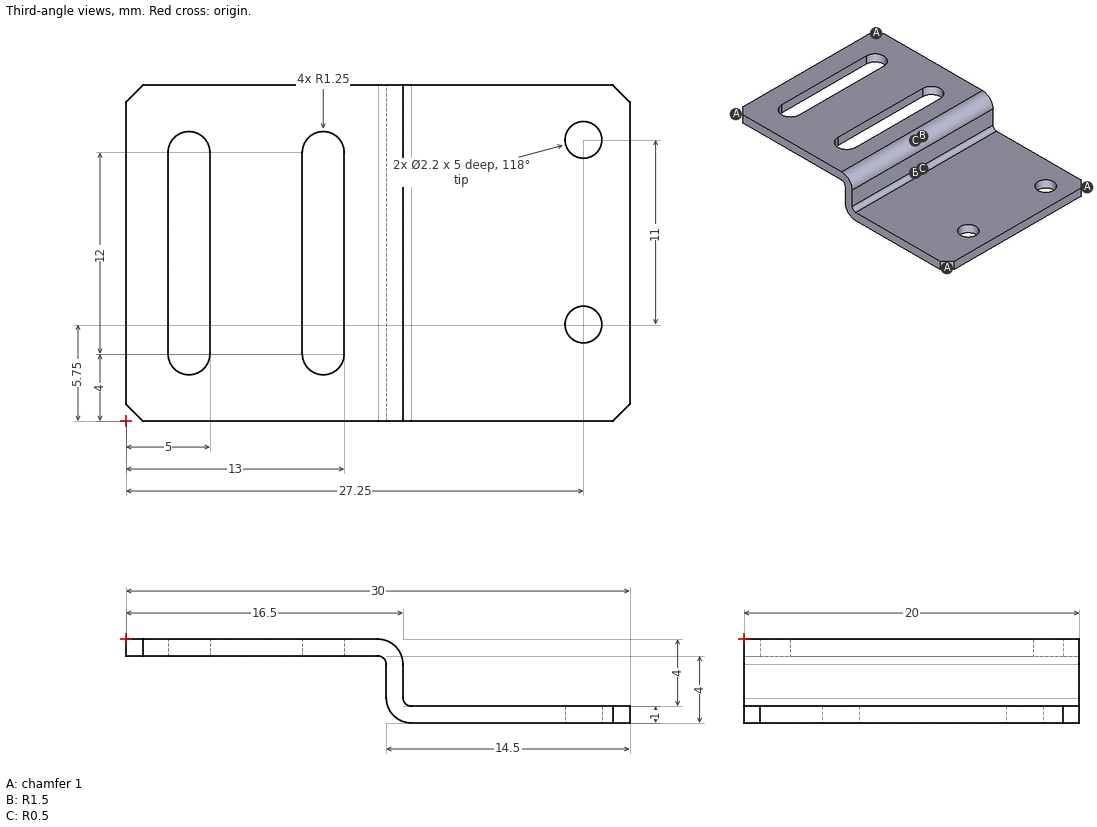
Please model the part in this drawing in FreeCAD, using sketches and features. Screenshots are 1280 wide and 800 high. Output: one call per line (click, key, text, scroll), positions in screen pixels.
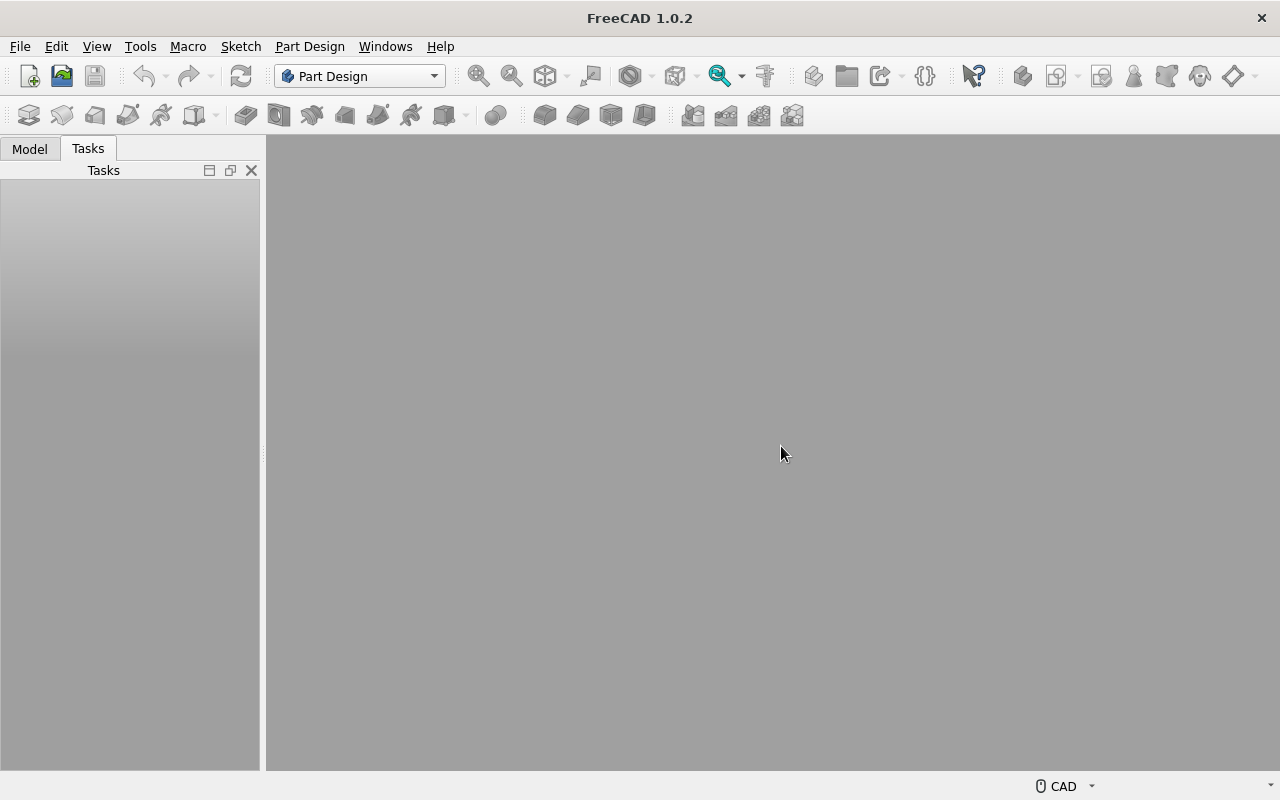
click(29, 76)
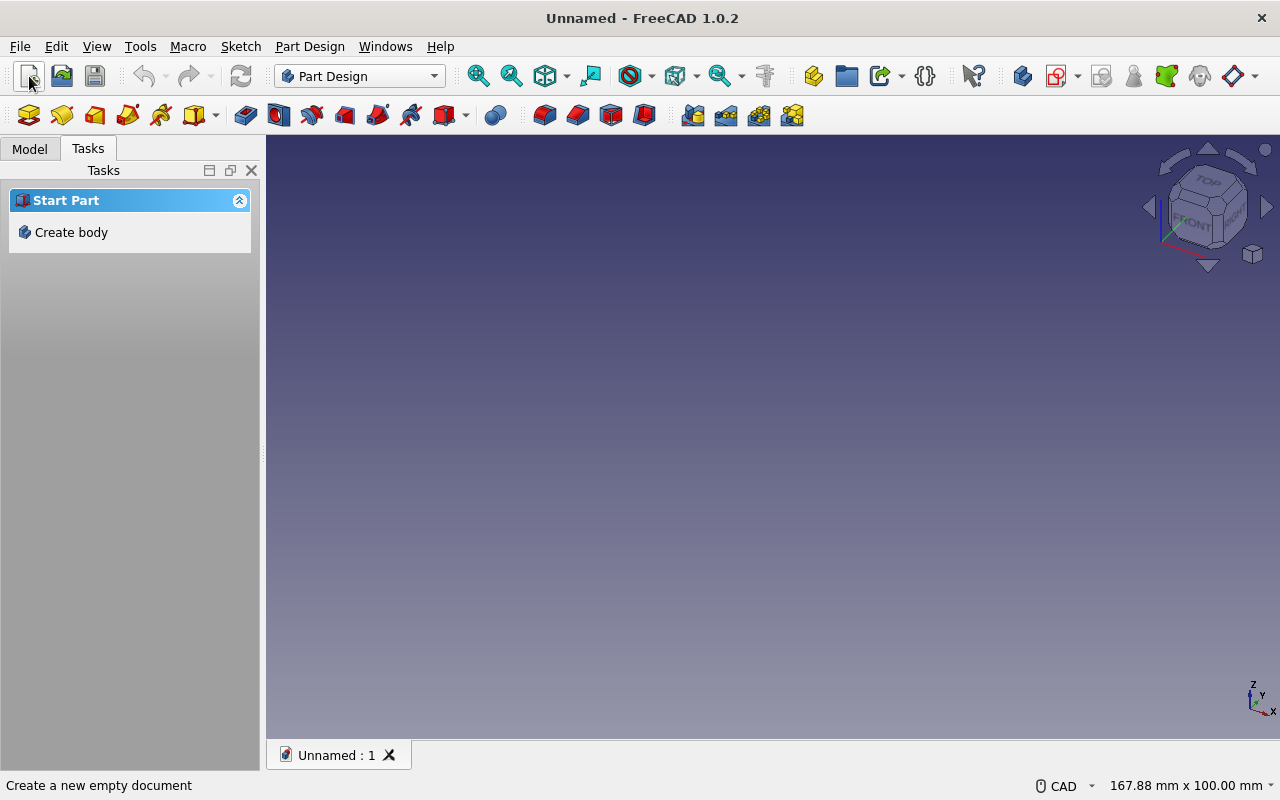
click(1056, 76)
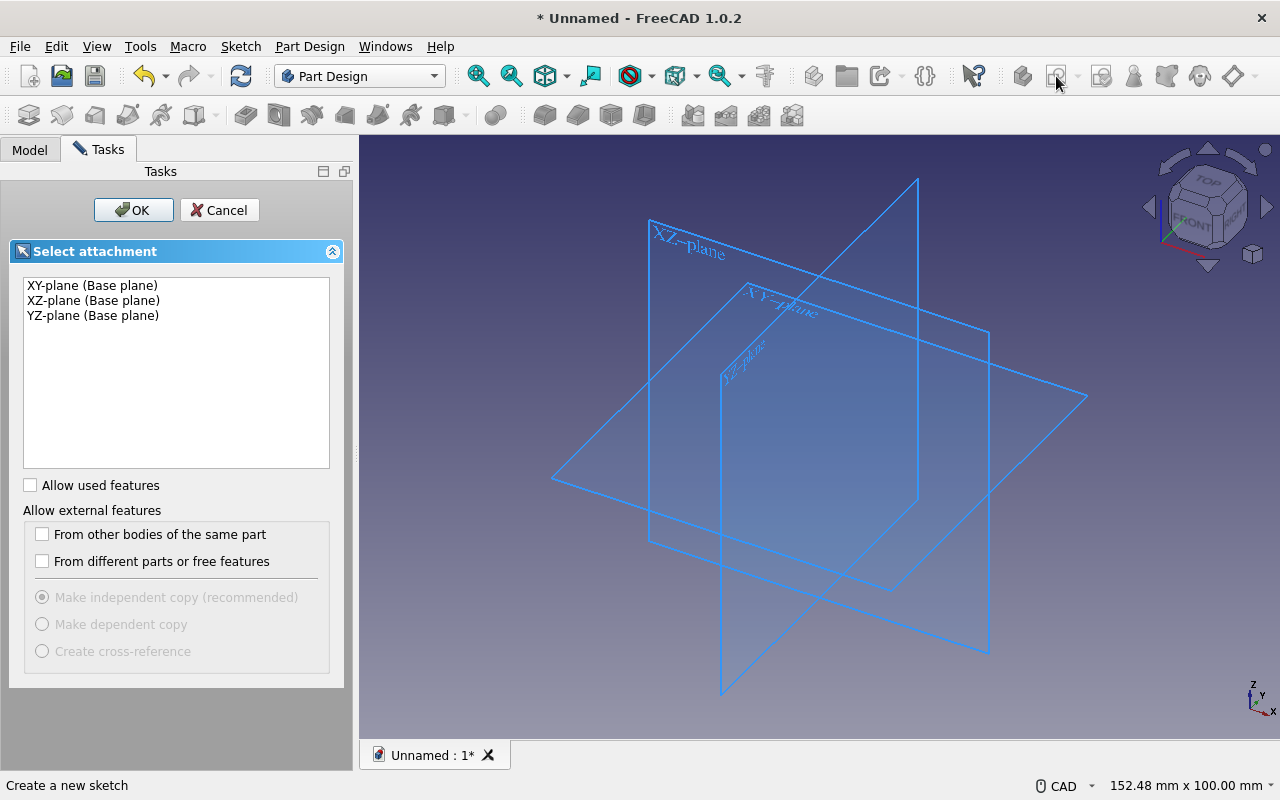
click(84, 300)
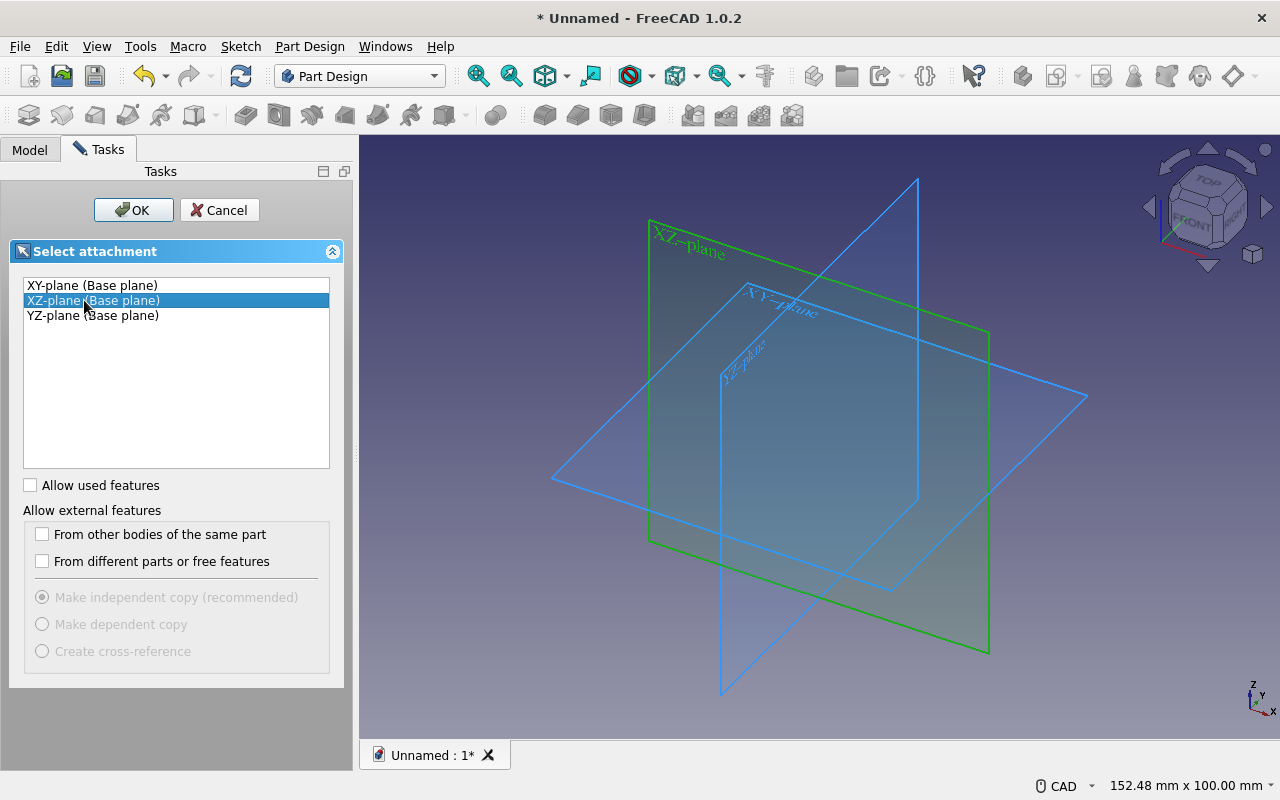
click(134, 210)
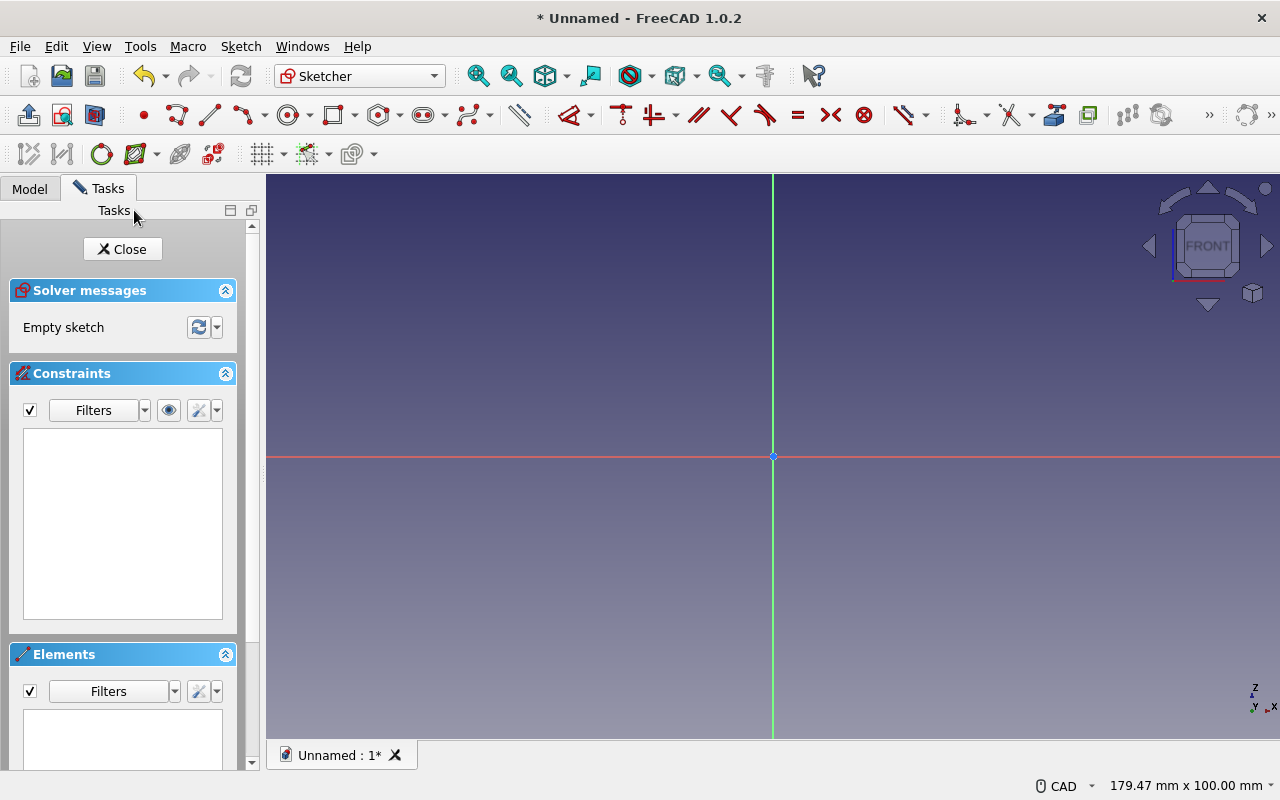
scroll(924, 477, up, 6)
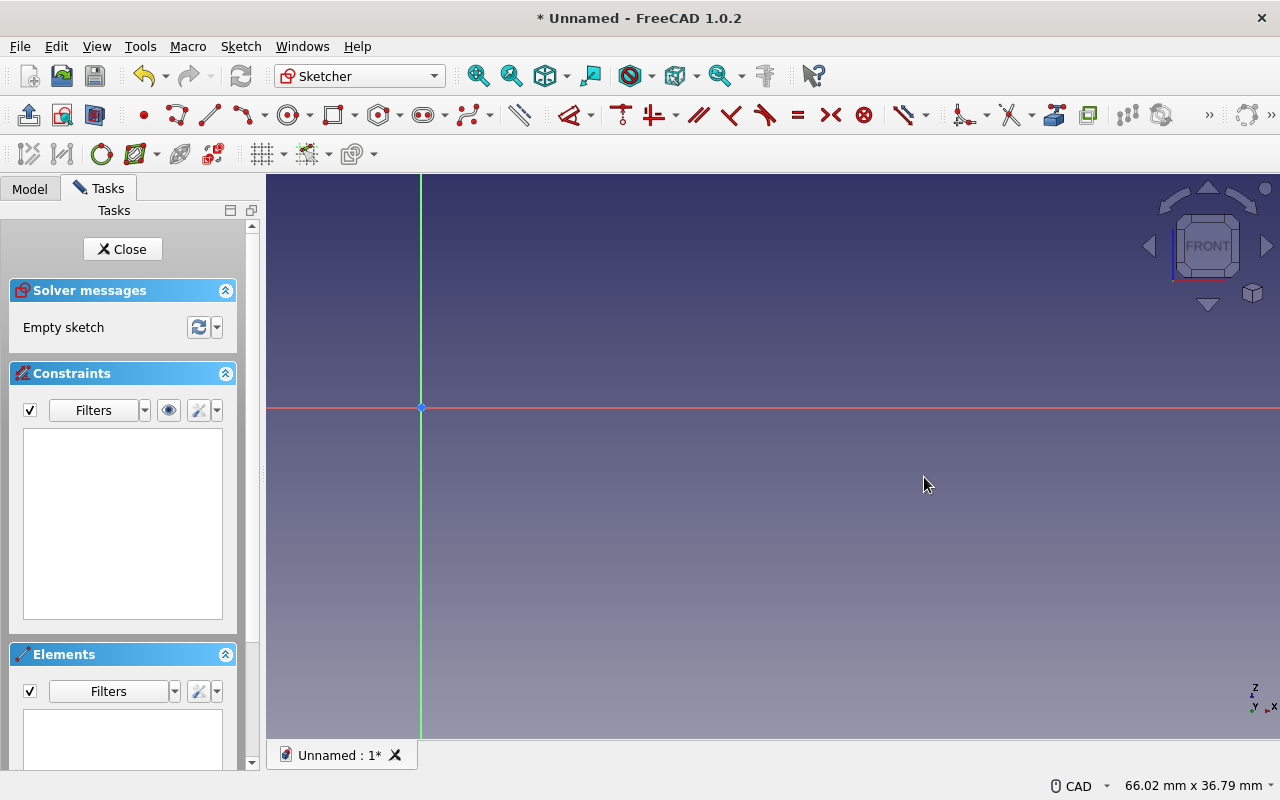
click(177, 116)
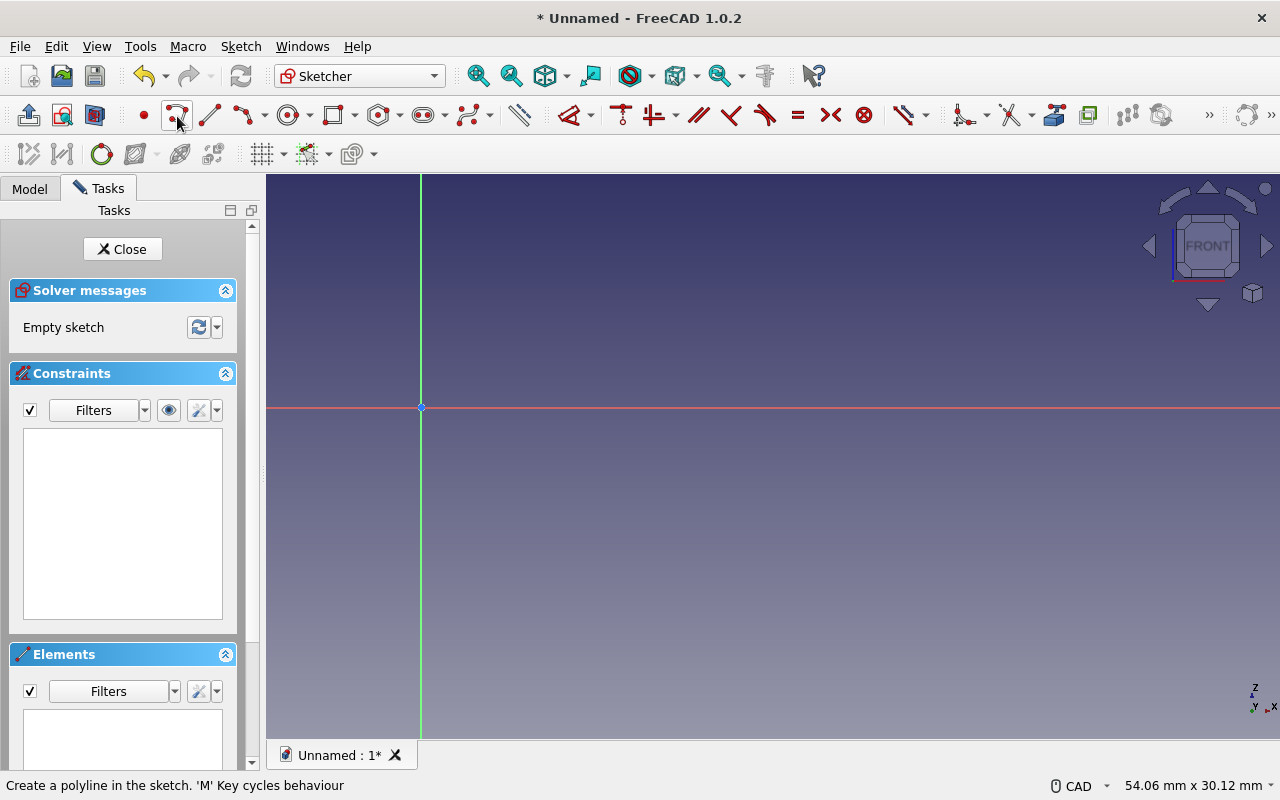
click(421, 408)
click(731, 417)
click(731, 483)
click(984, 483)
click(984, 501)
click(712, 501)
click(712, 426)
click(430, 426)
click(421, 408)
key(Escape)
key(Escape)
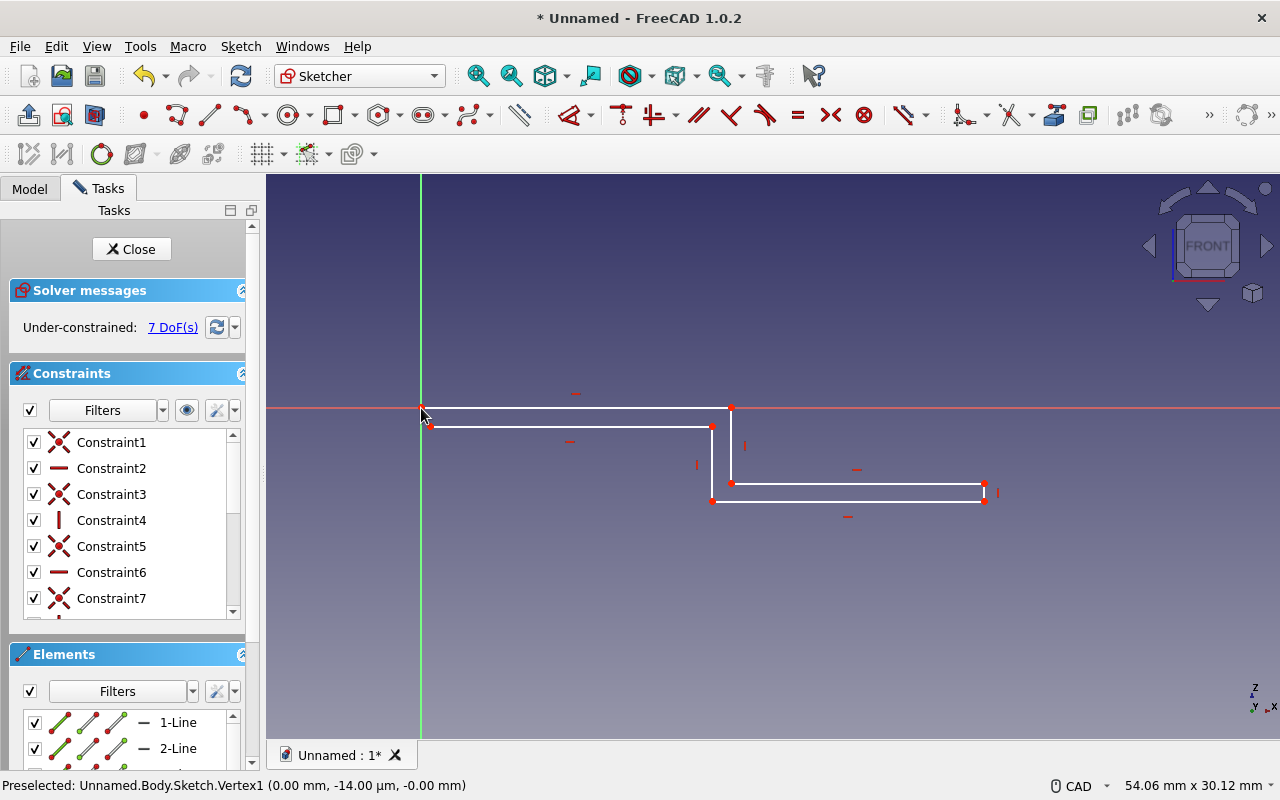
scroll(425, 415, up, 3)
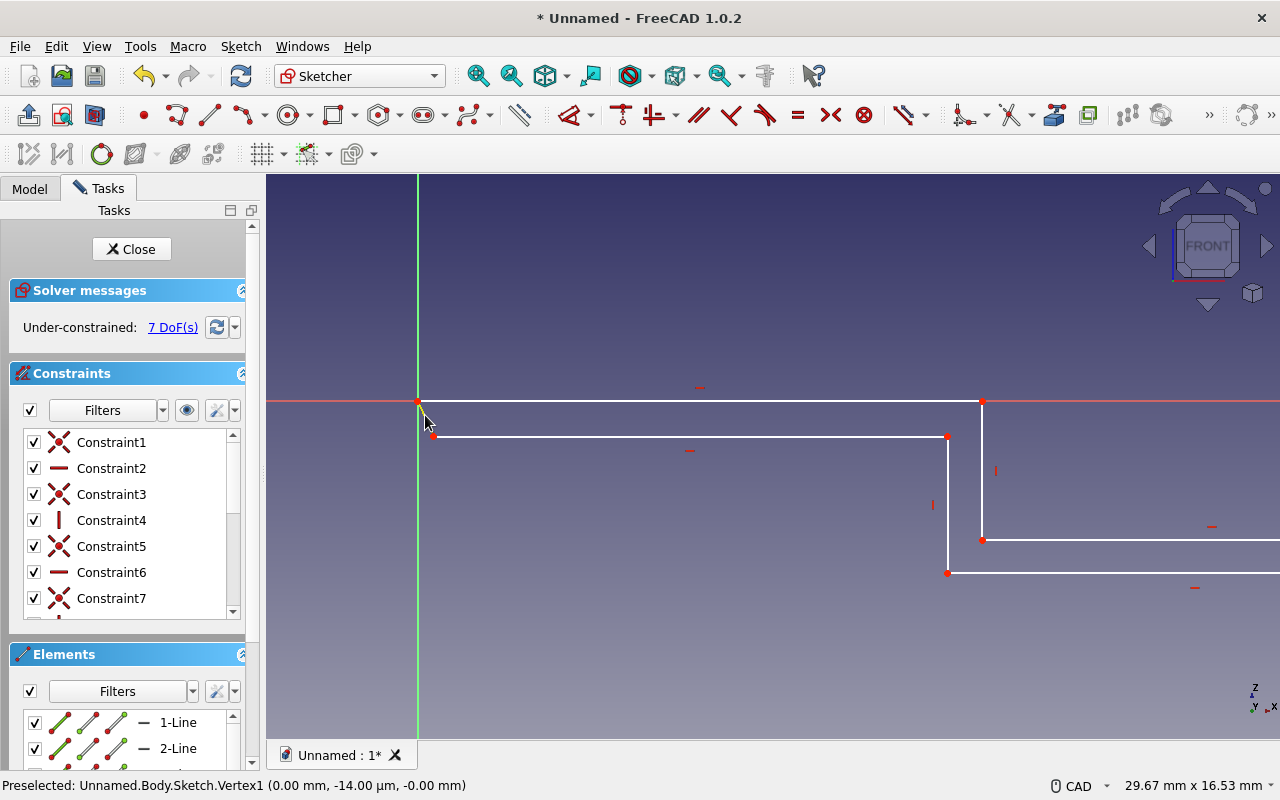
click(424, 415)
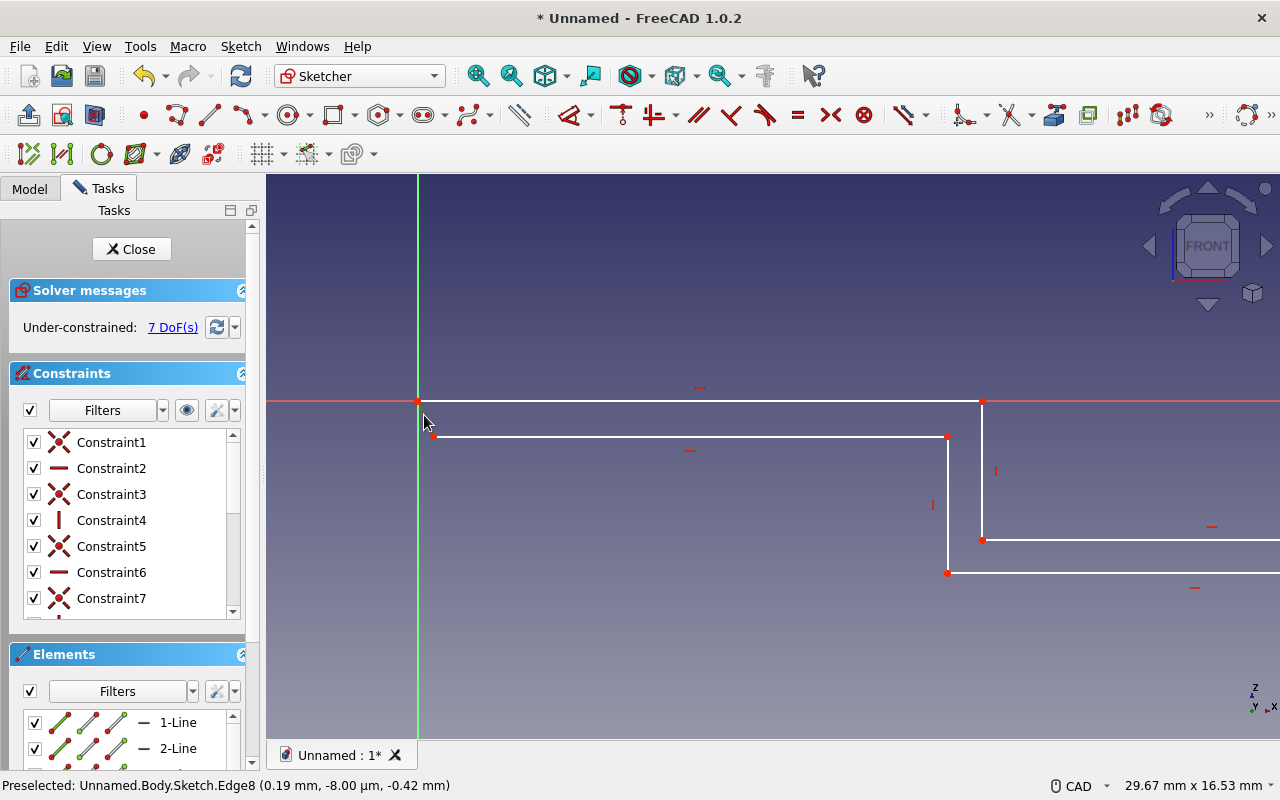
click(676, 116)